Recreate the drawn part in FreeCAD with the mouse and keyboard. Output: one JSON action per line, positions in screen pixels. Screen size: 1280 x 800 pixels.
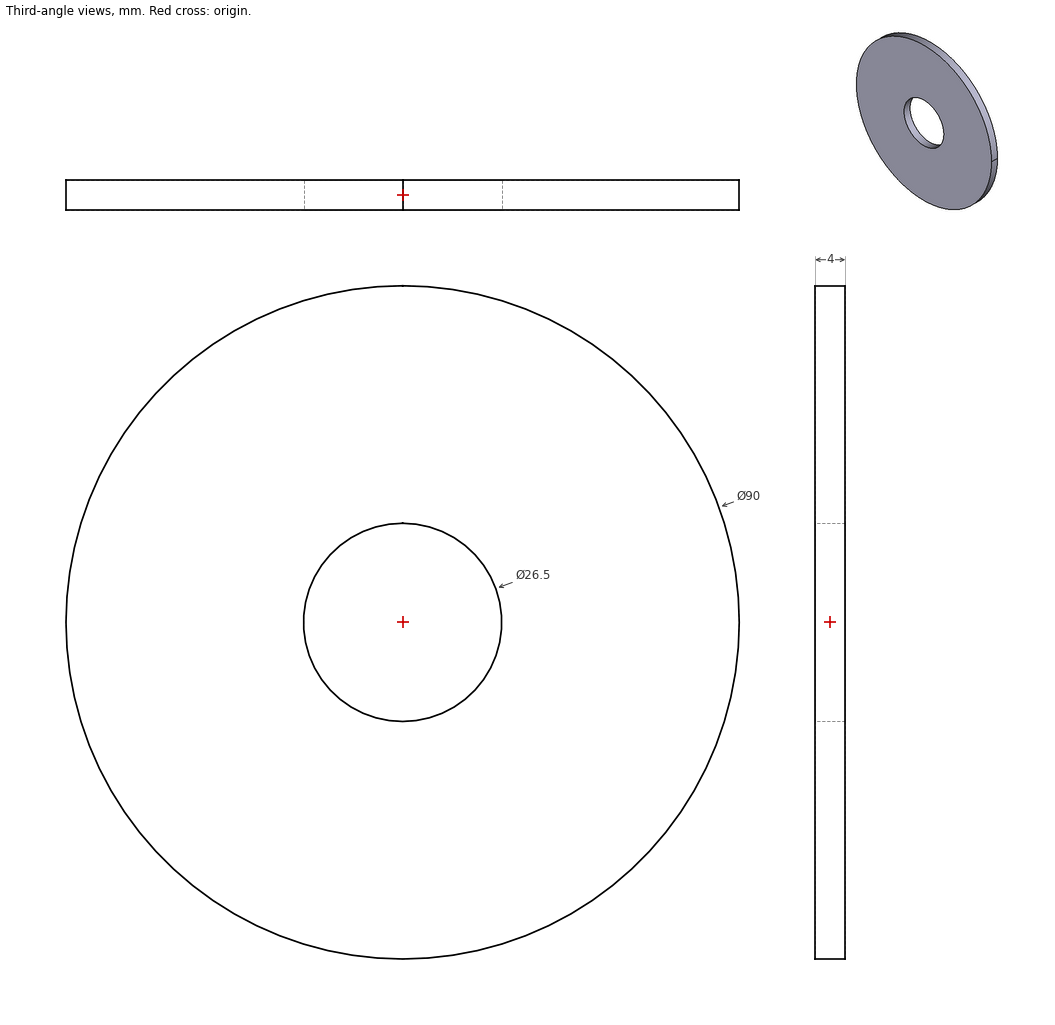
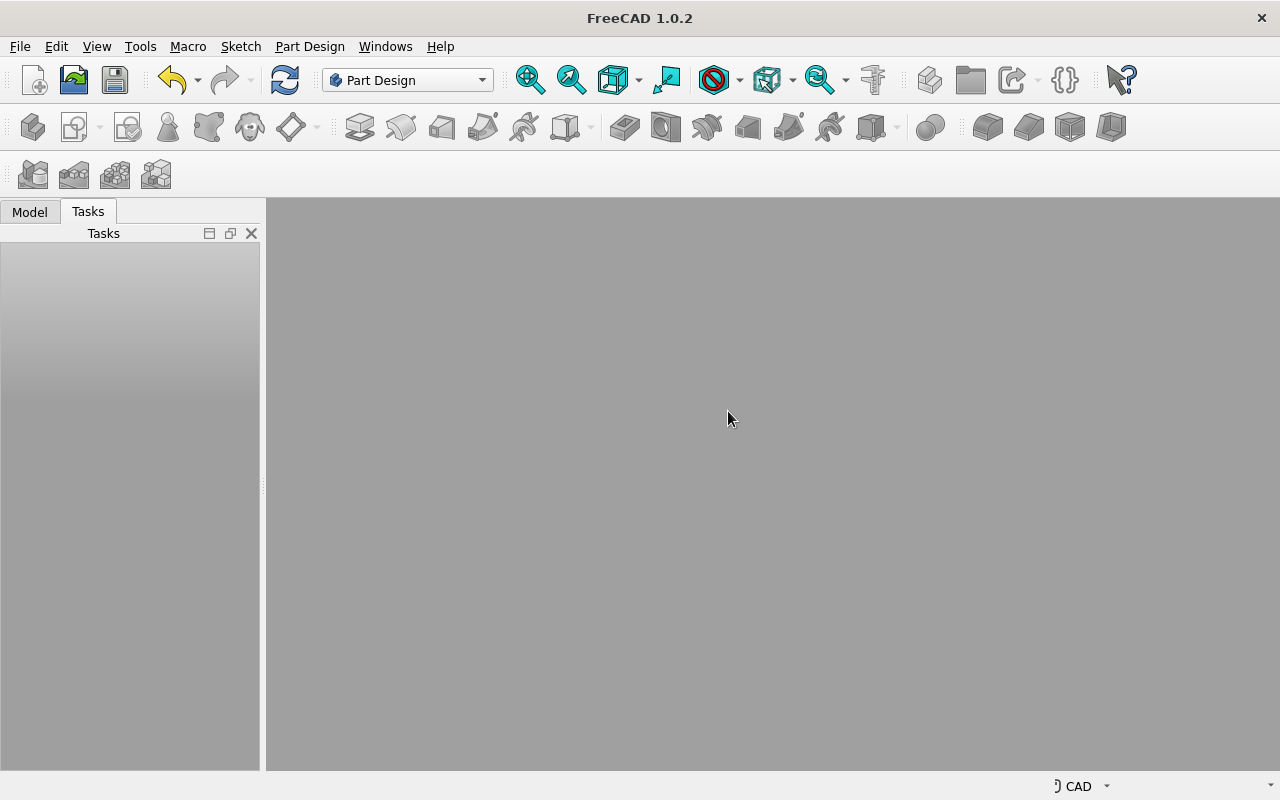
{"action": "left_click", "coordinate": [33, 80]}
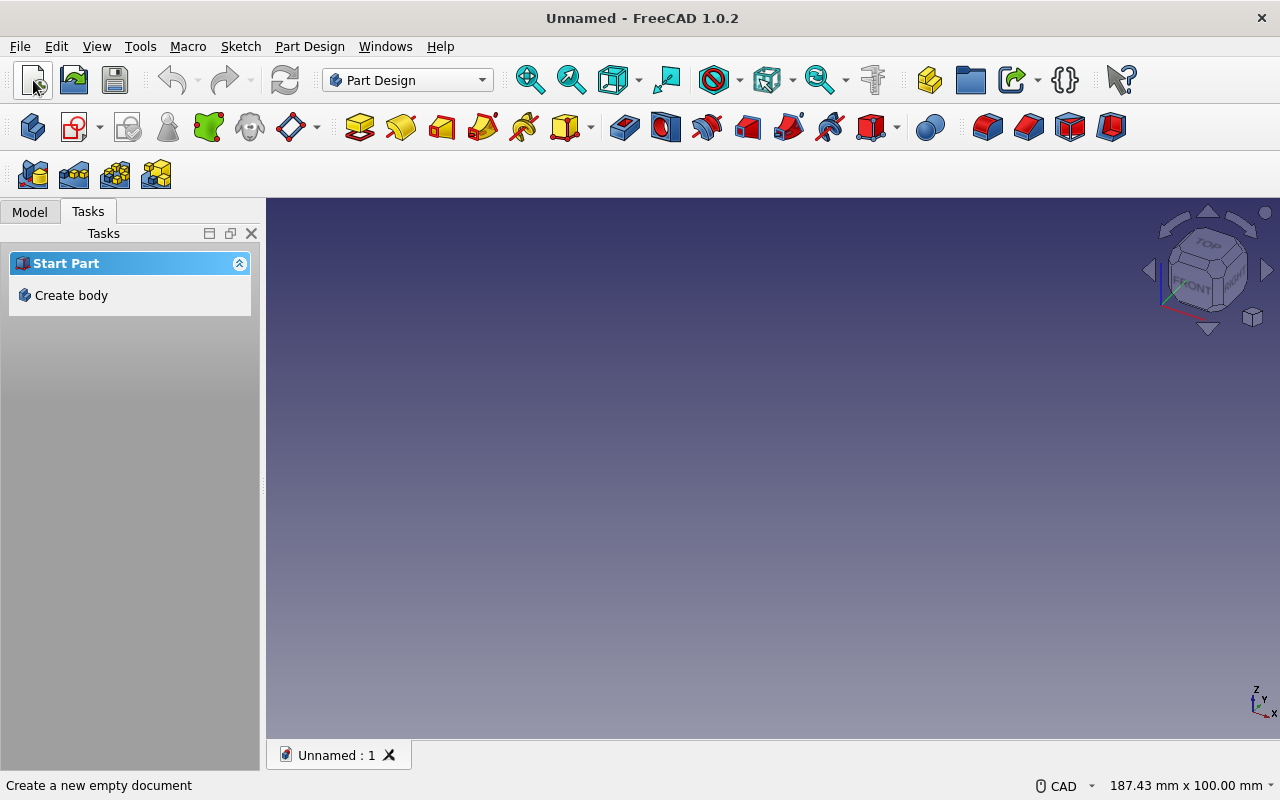
{"action": "left_click", "coordinate": [74, 128]}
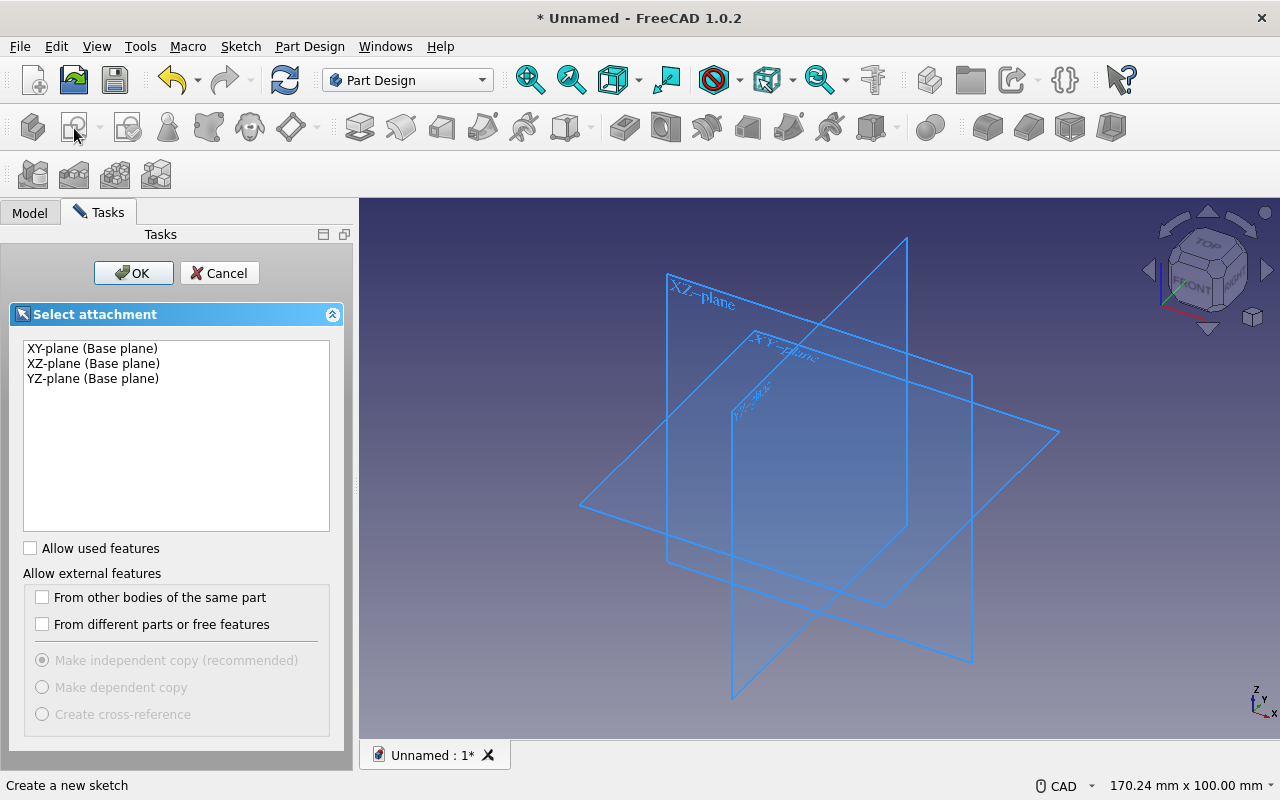
{"action": "left_click", "coordinate": [84, 364]}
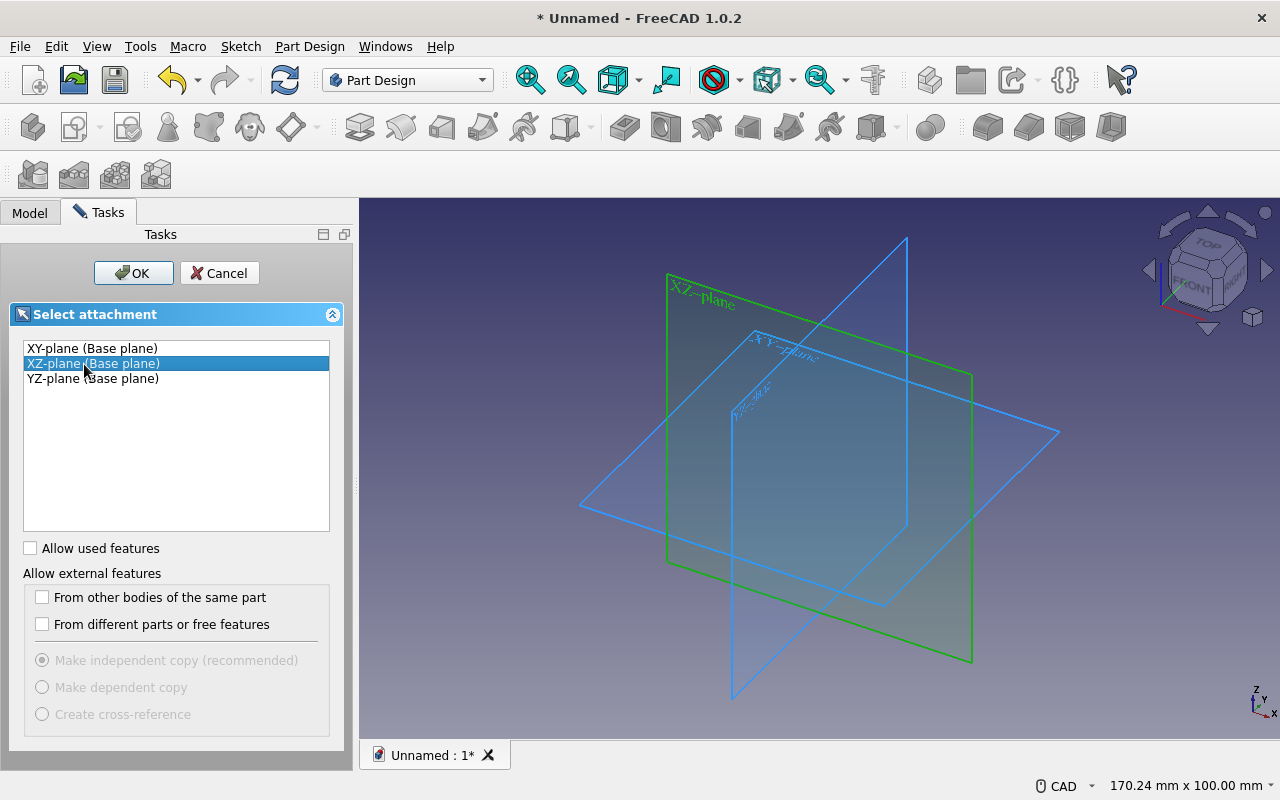
{"action": "left_click", "coordinate": [134, 273]}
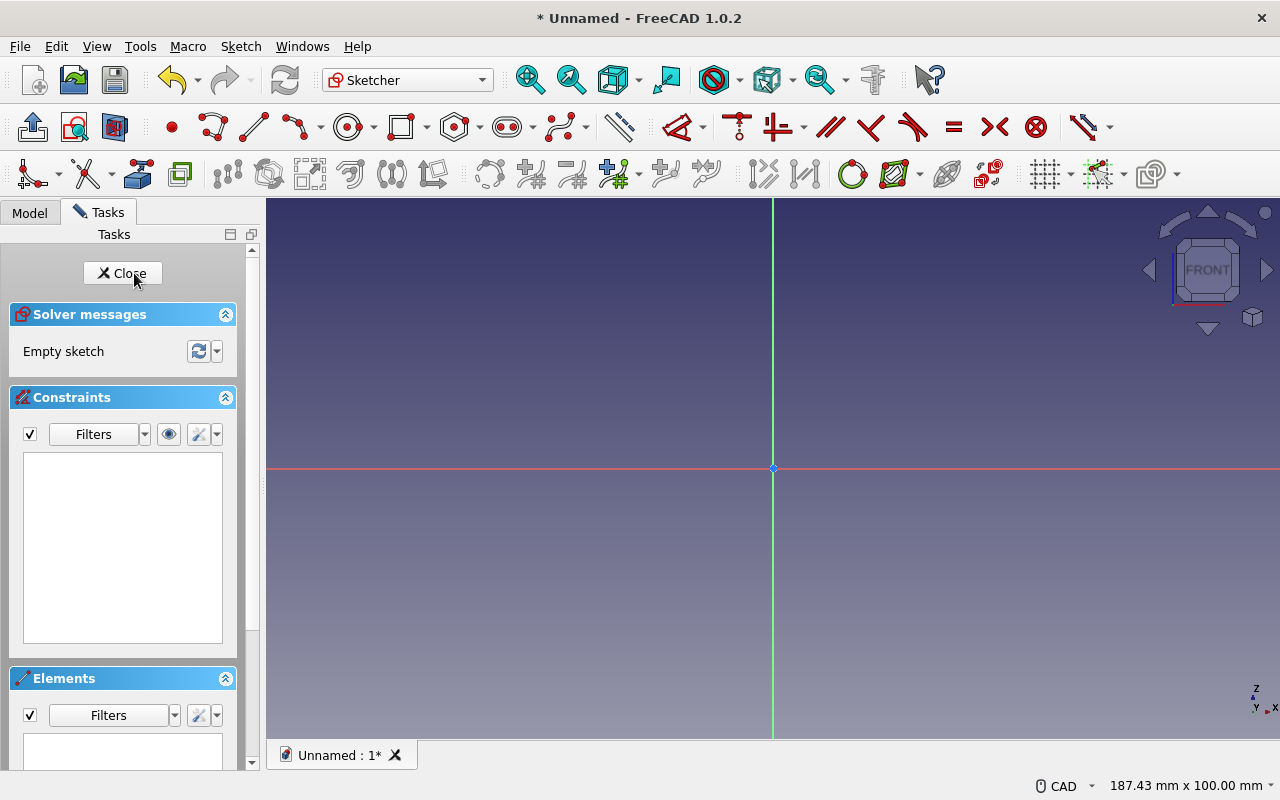
{"action": "scroll", "coordinate": [565, 468], "scroll_direction": "down", "scroll_amount": 2}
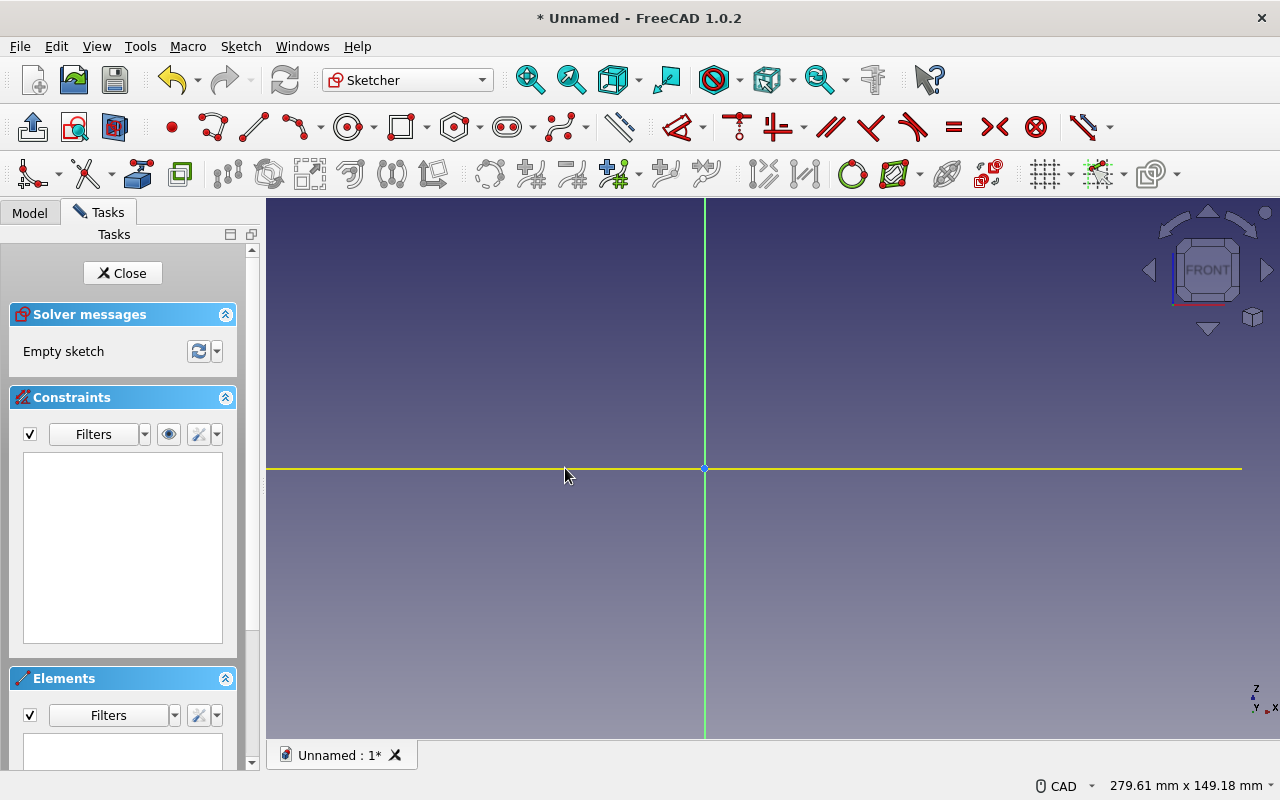
{"action": "key", "text": "g c"}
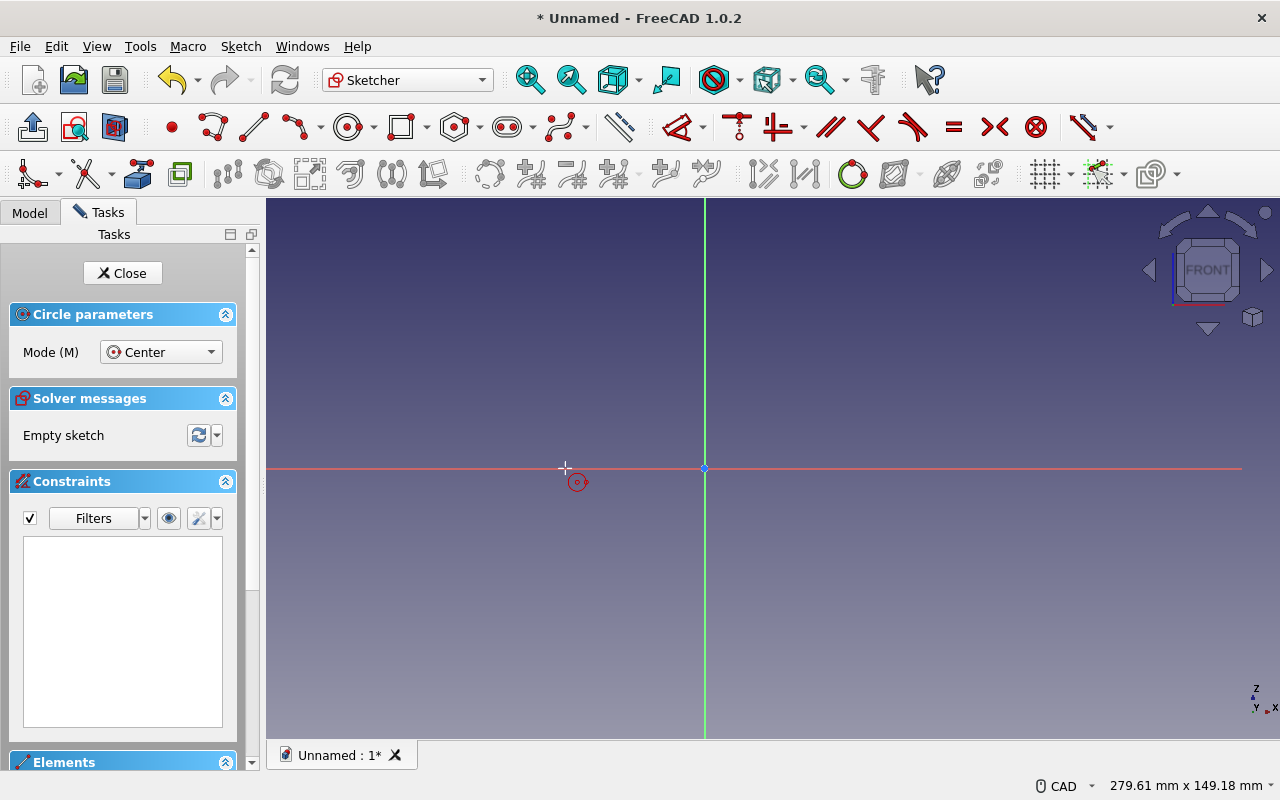
{"action": "left_click", "coordinate": [705, 468]}
{"action": "mouse_move", "coordinate": [820, 353]}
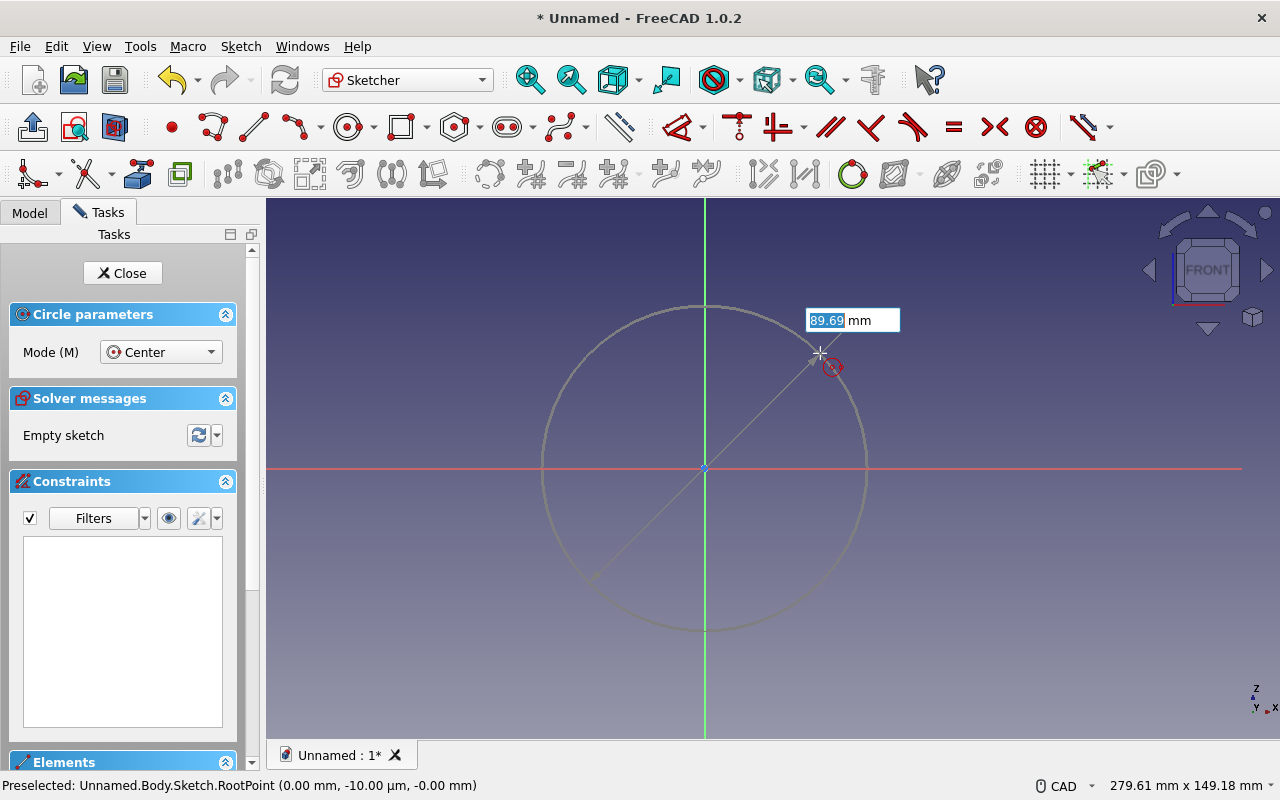
{"action": "type", "text": "90"}
{"action": "key", "text": "Return"}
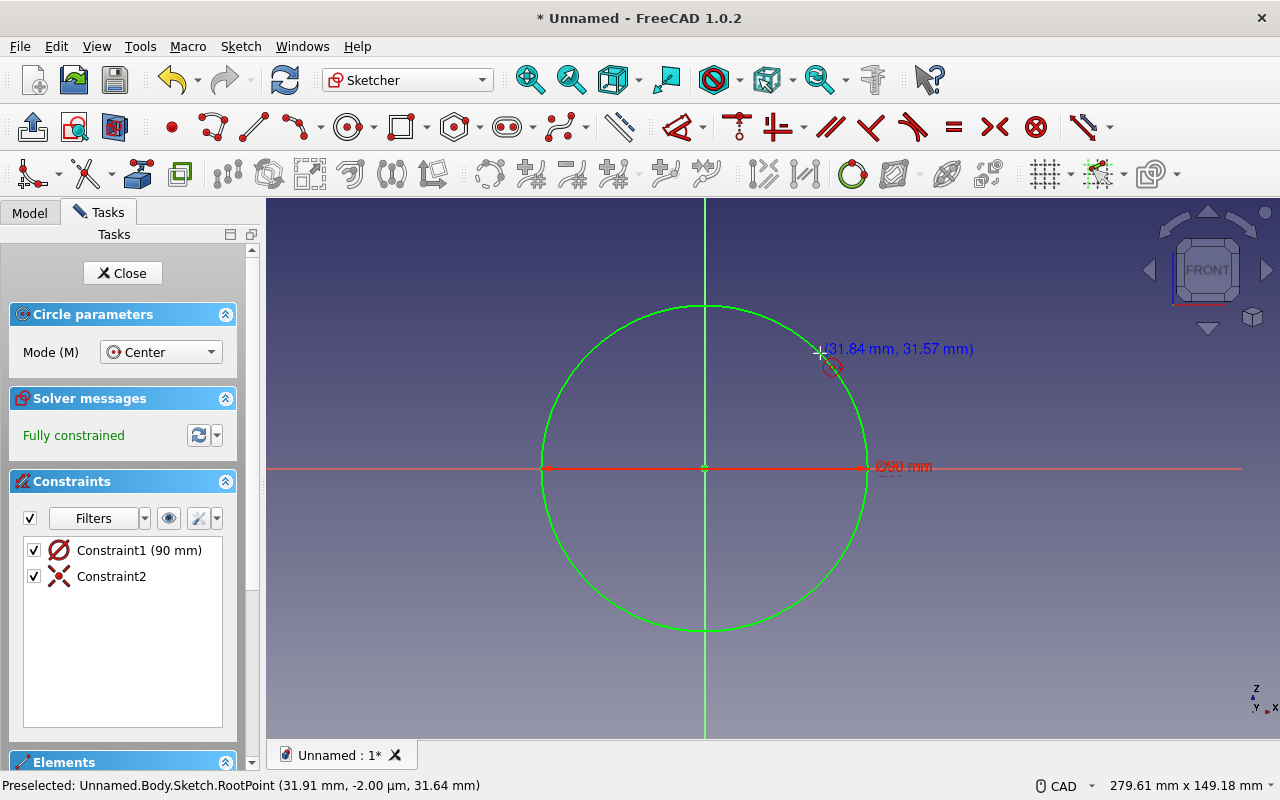
{"action": "left_click", "coordinate": [705, 468]}
{"action": "mouse_move", "coordinate": [739, 435]}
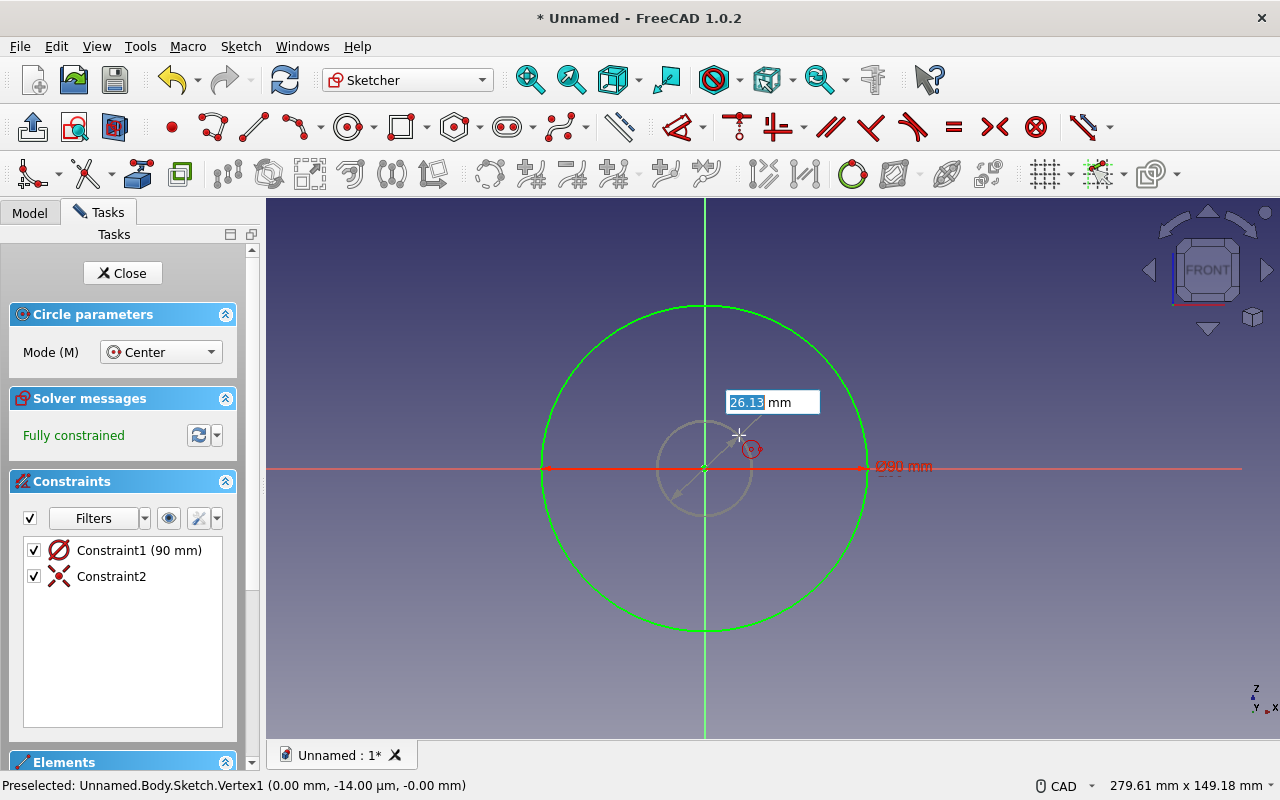
{"action": "type", "text": "26.5"}
{"action": "key", "text": "Return"}
{"action": "key", "text": "Escape"}